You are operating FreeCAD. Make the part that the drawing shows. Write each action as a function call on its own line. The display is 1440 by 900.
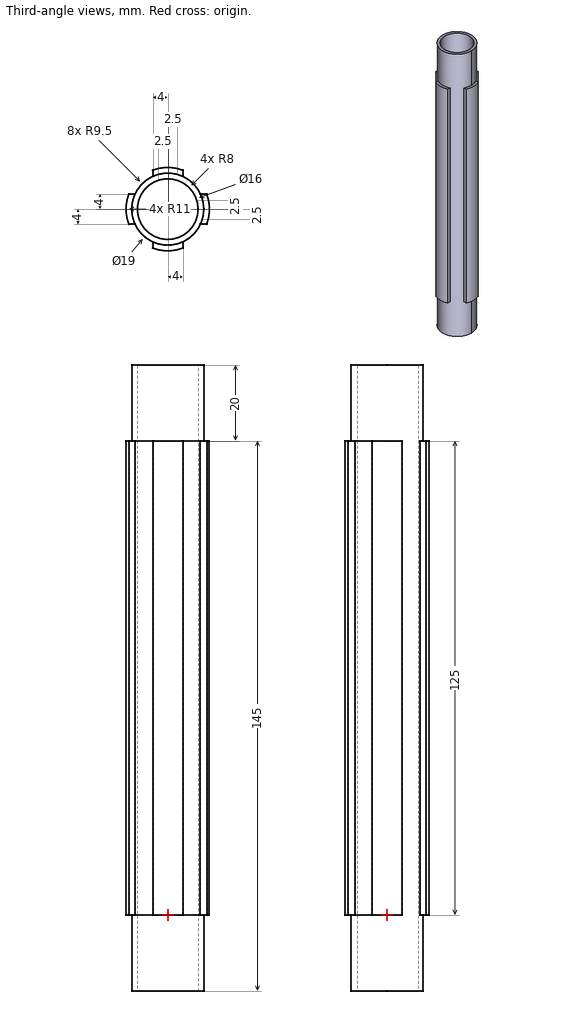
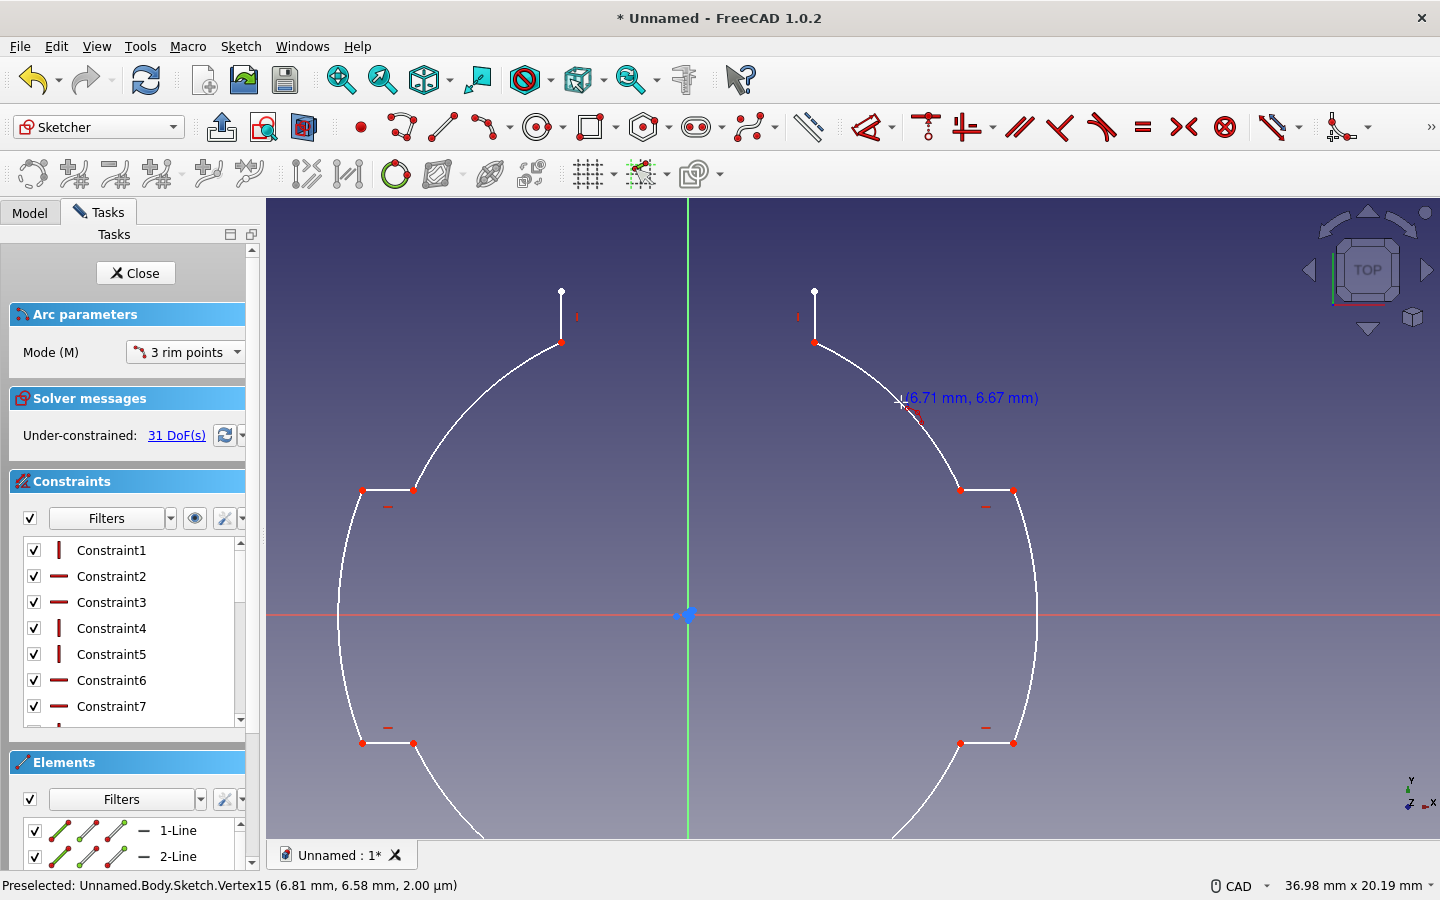
click(815, 291)
click(561, 291)
click(714, 267)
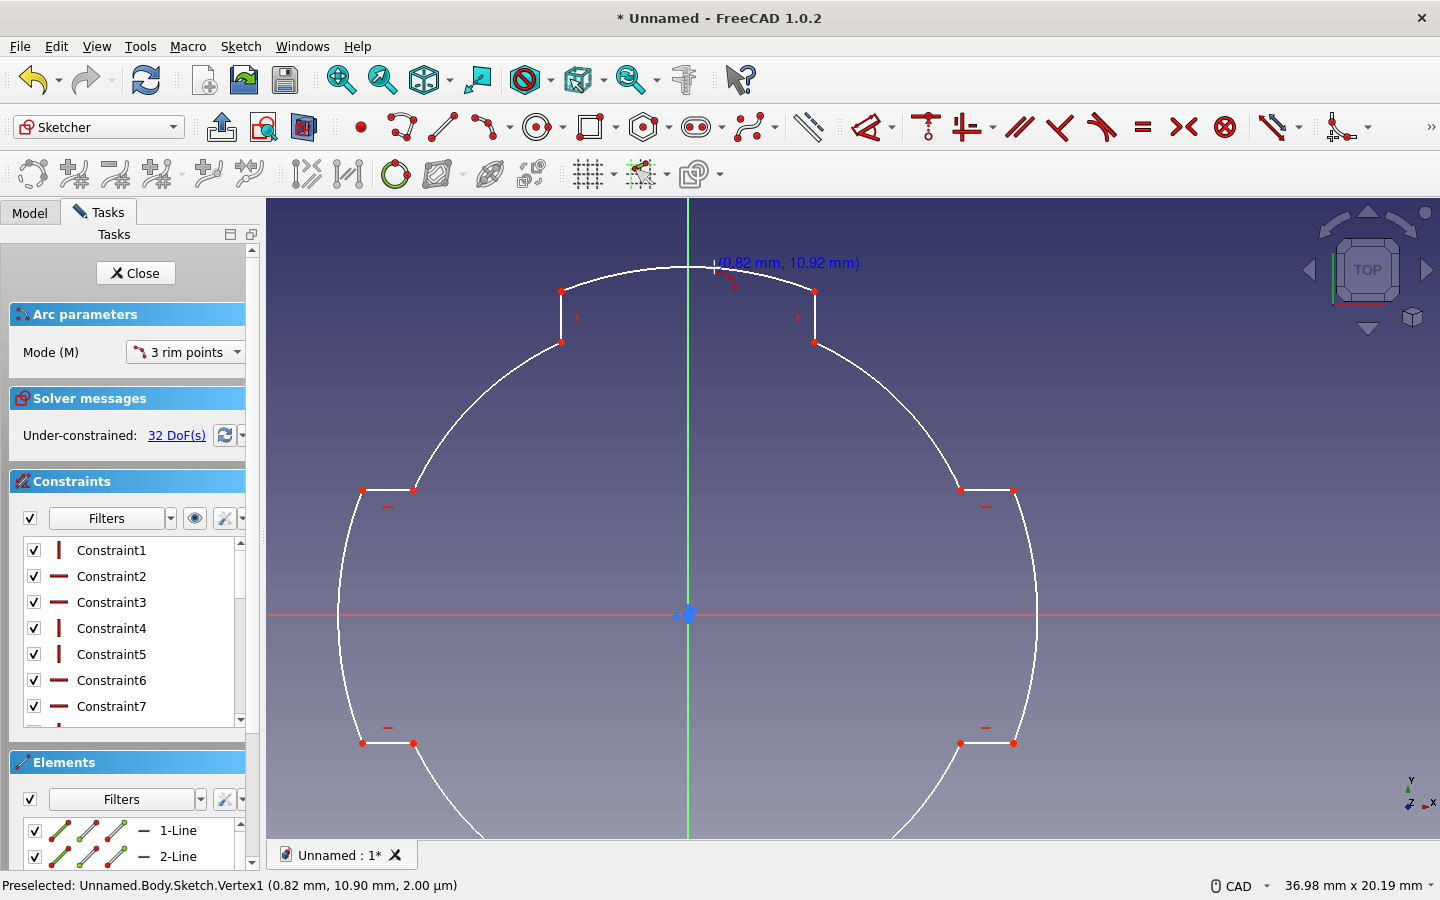
click(443, 128)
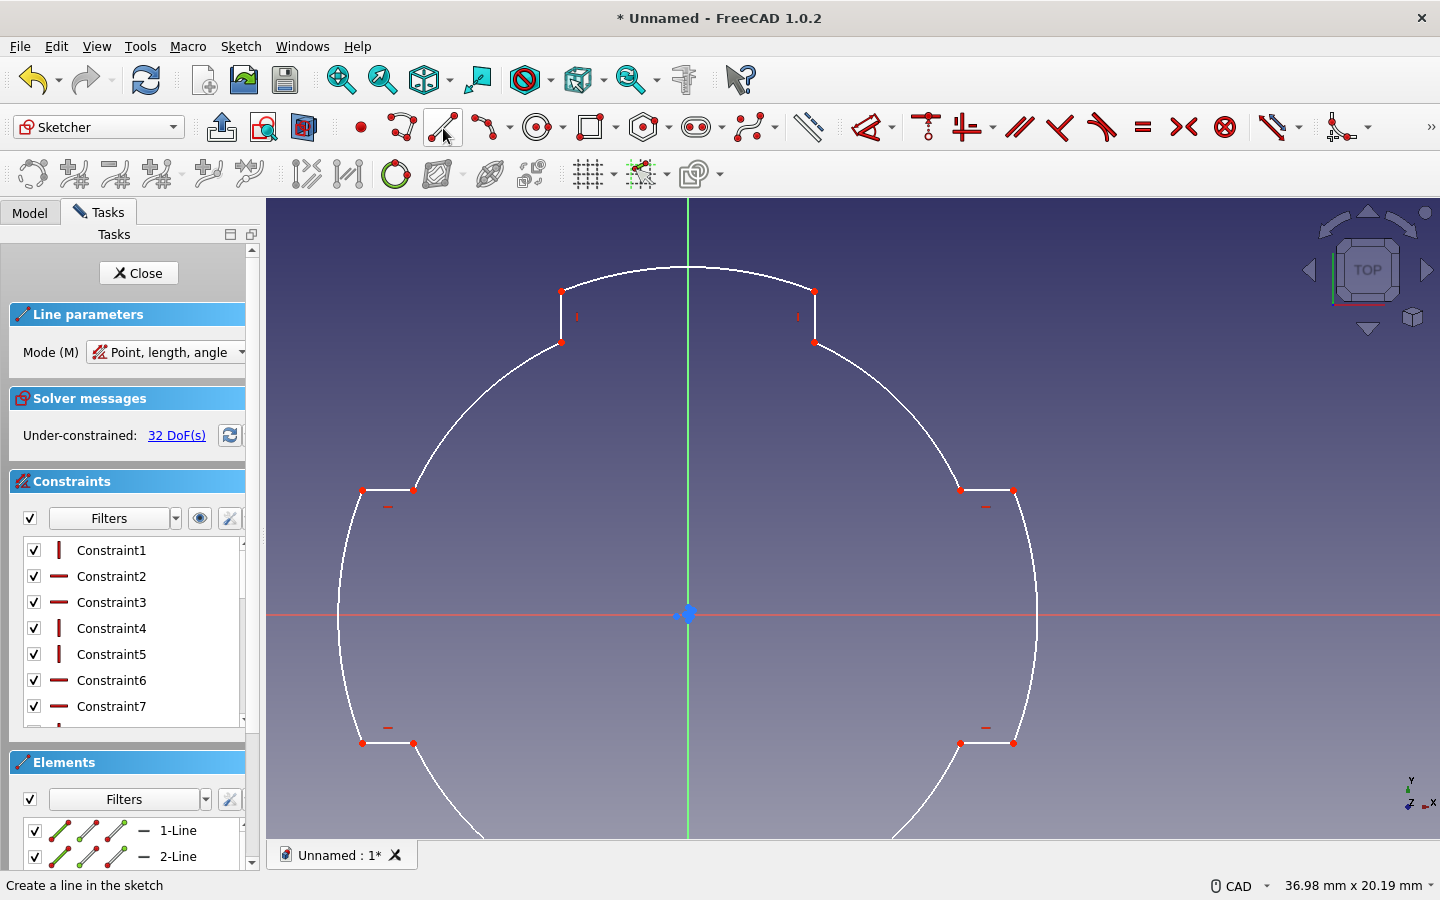
click(608, 374)
click(608, 324)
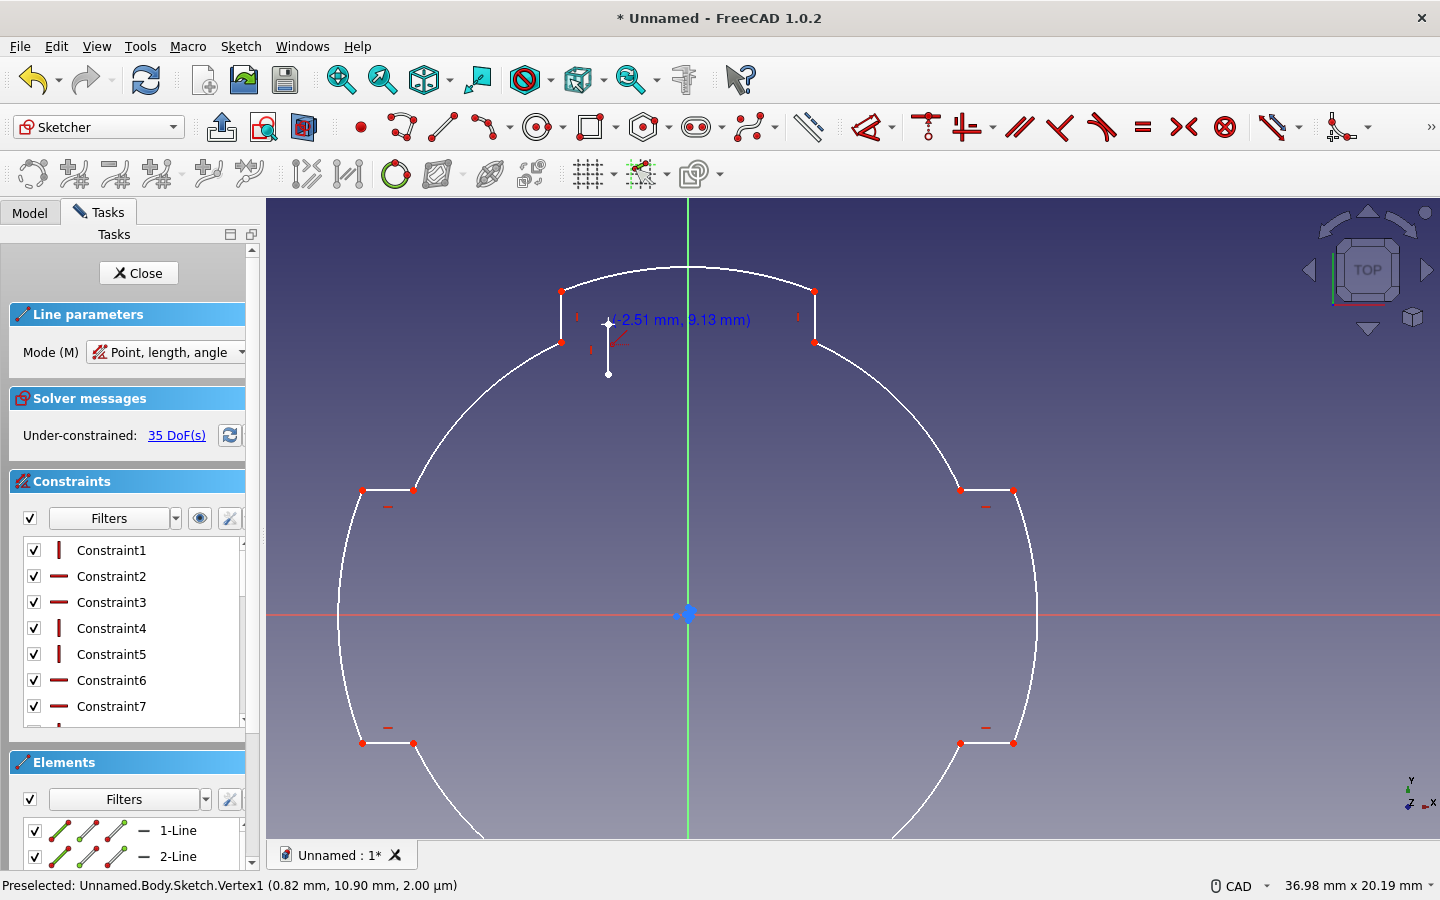
click(767, 324)
click(767, 374)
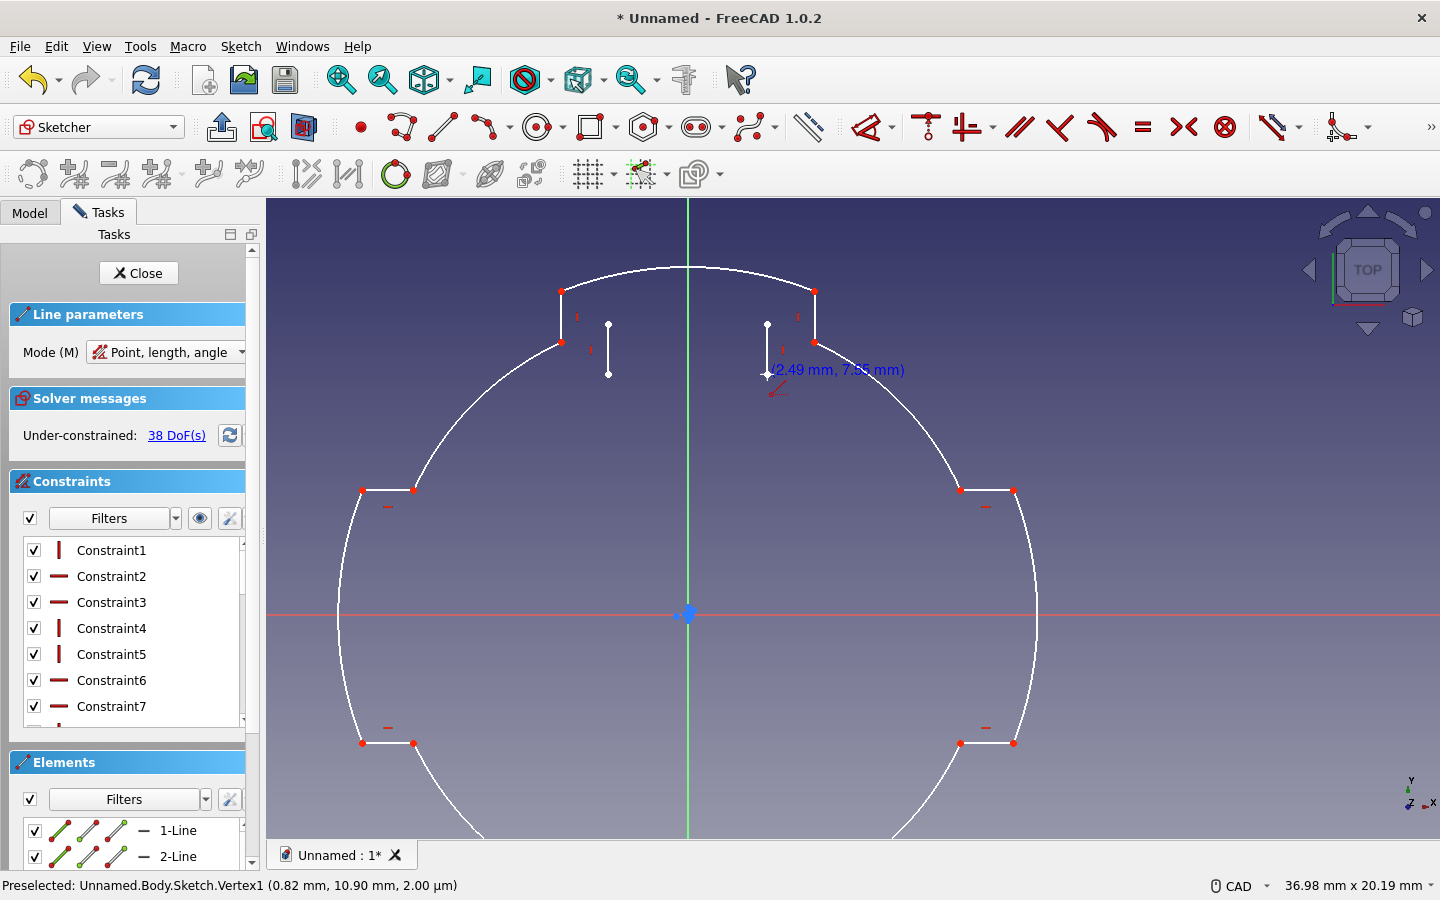
click(929, 535)
click(979, 535)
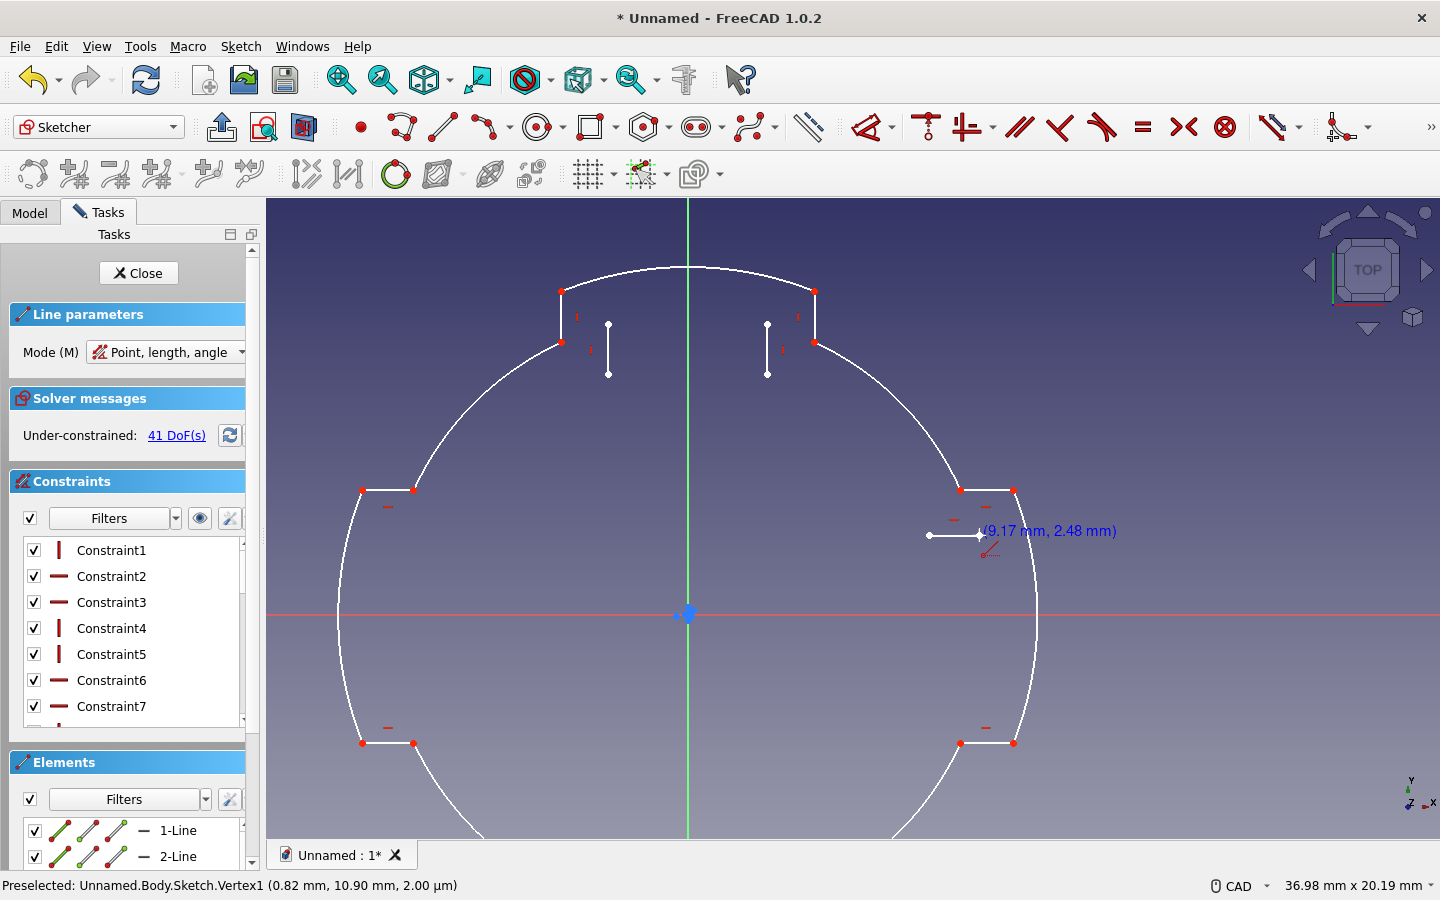
click(979, 694)
click(929, 694)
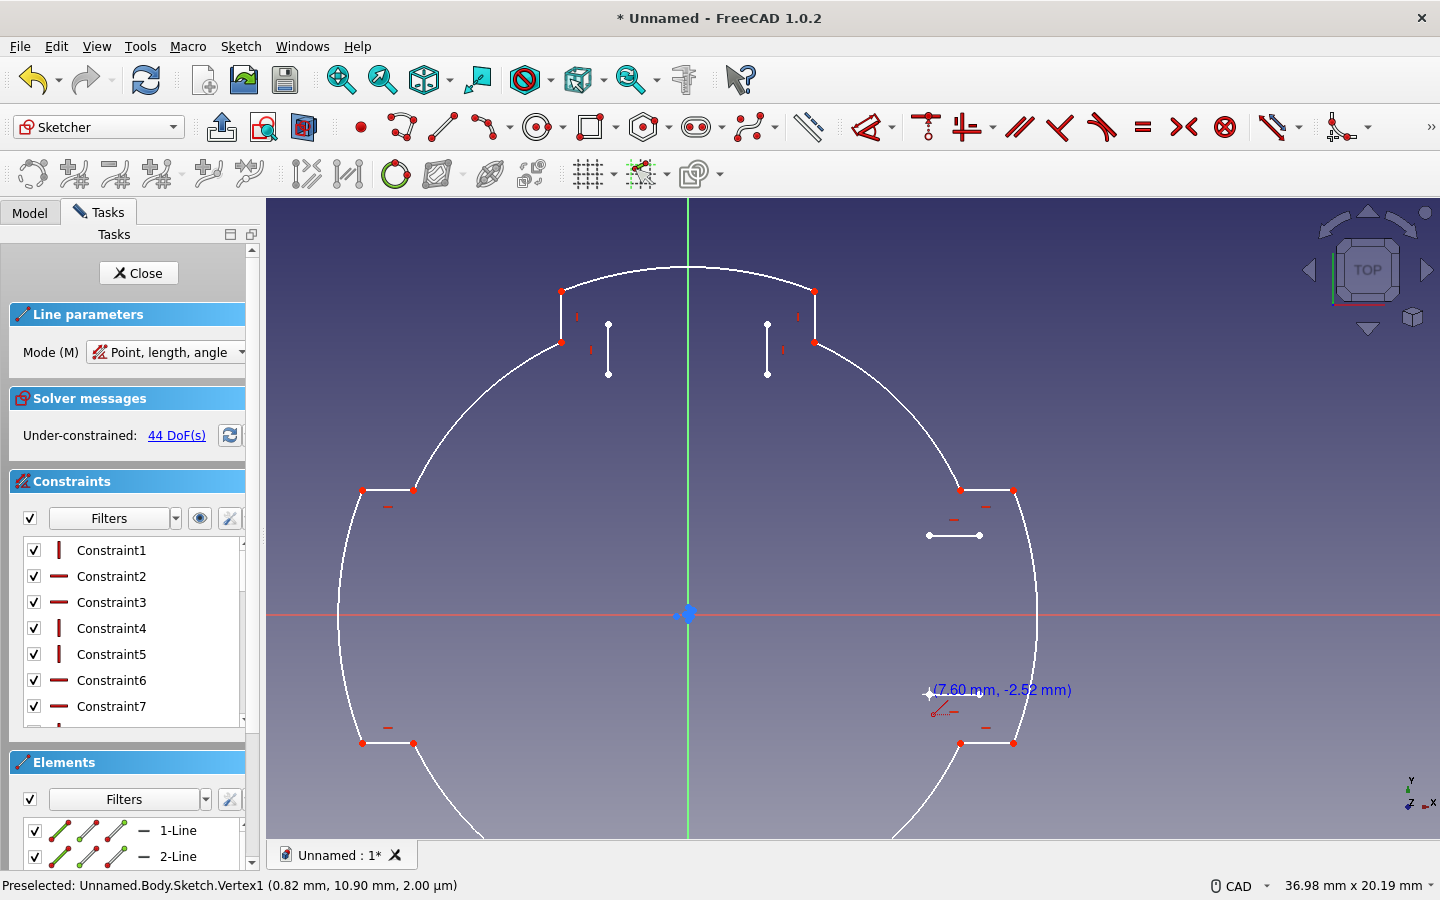
scroll(902, 401, down, 3)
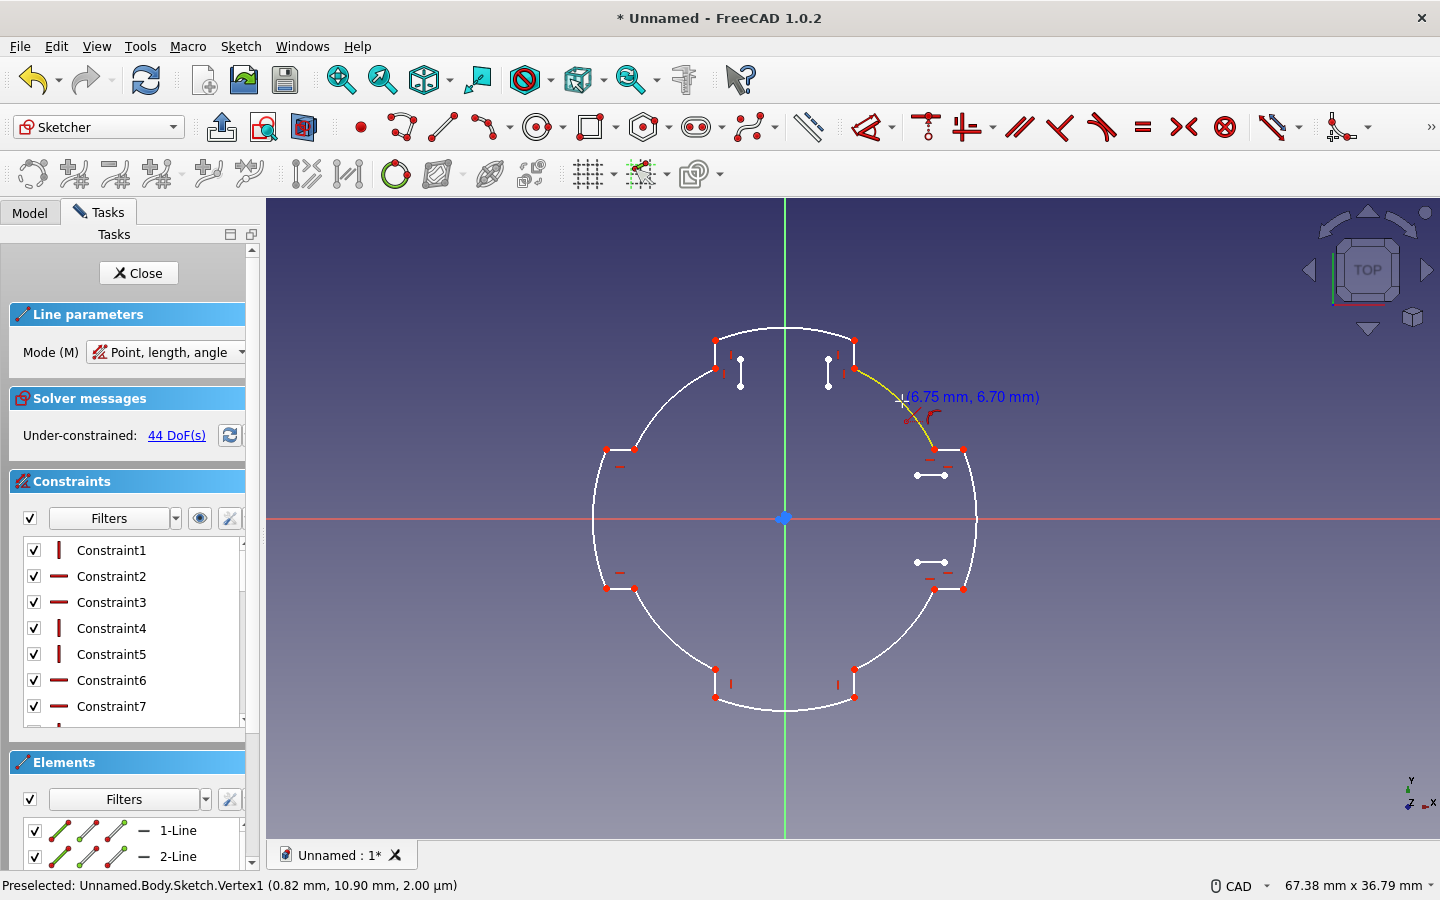
click(828, 651)
click(828, 678)